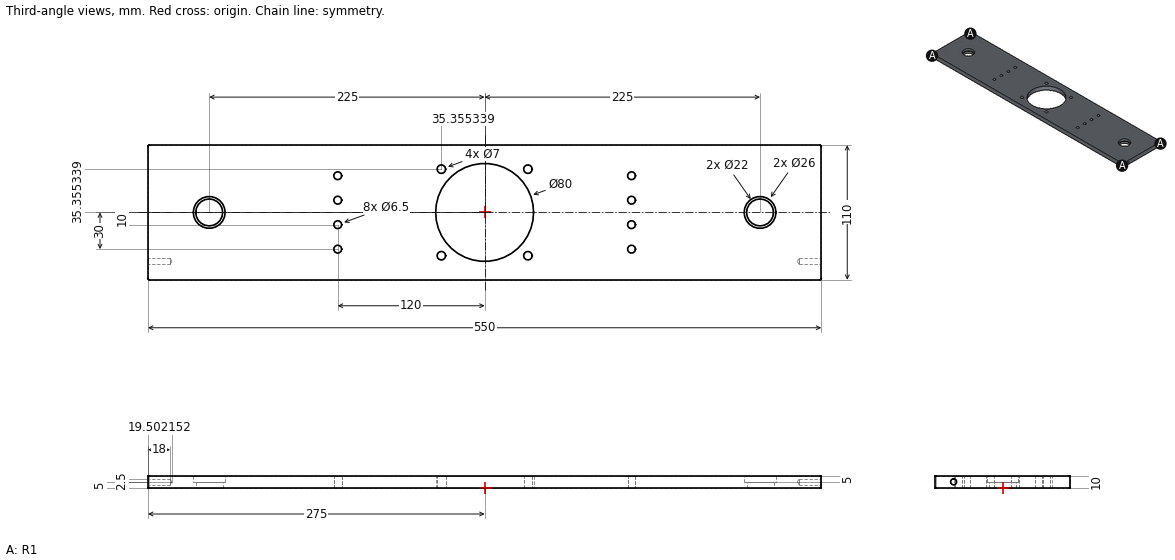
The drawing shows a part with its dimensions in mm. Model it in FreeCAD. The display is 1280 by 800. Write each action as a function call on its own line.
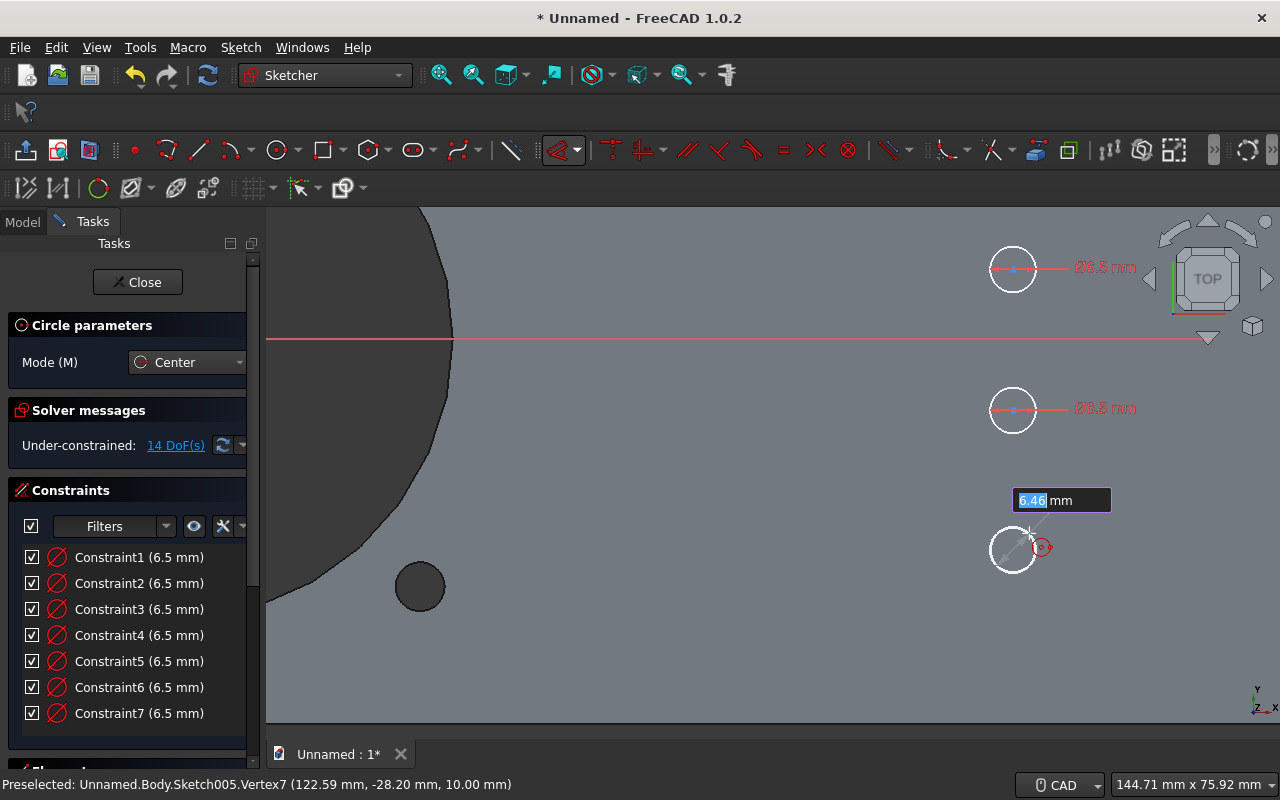
text(6.5)
key(Return)
key(Escape)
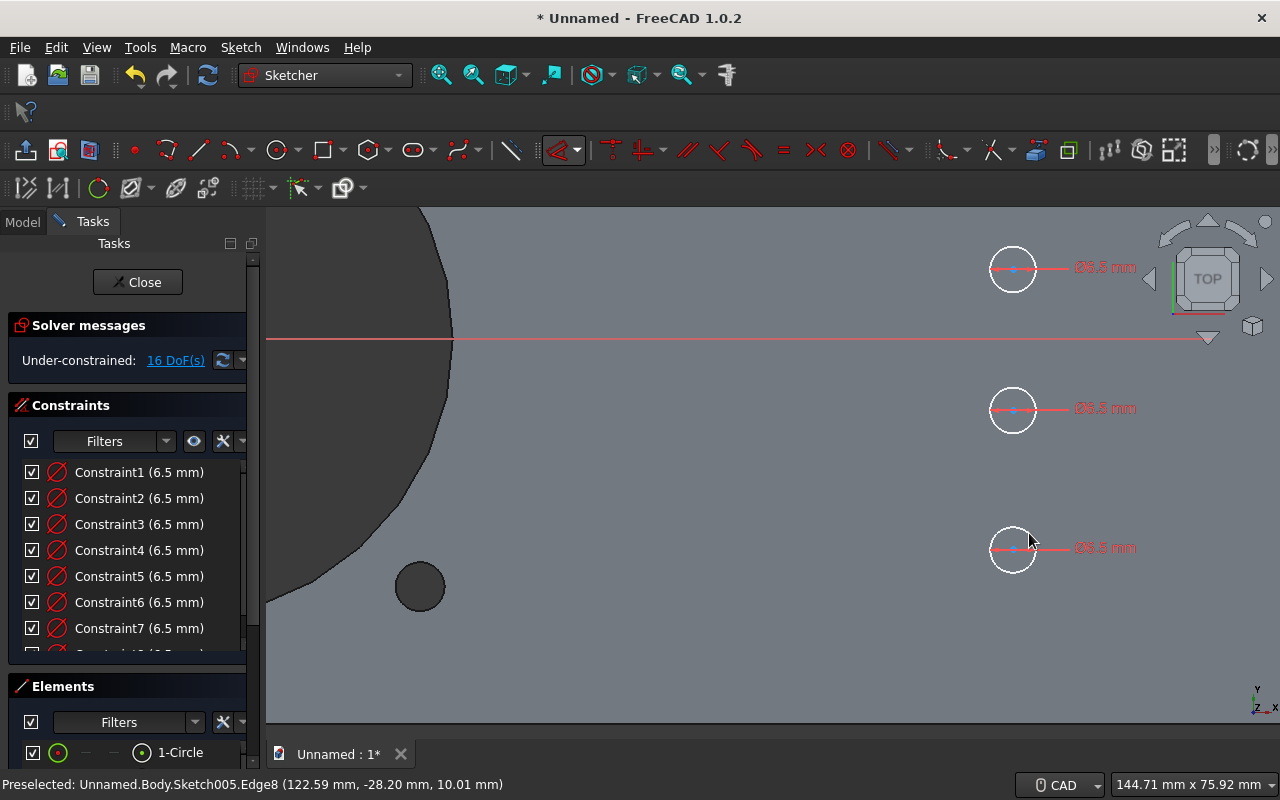
scroll(1014, 551, down, 5)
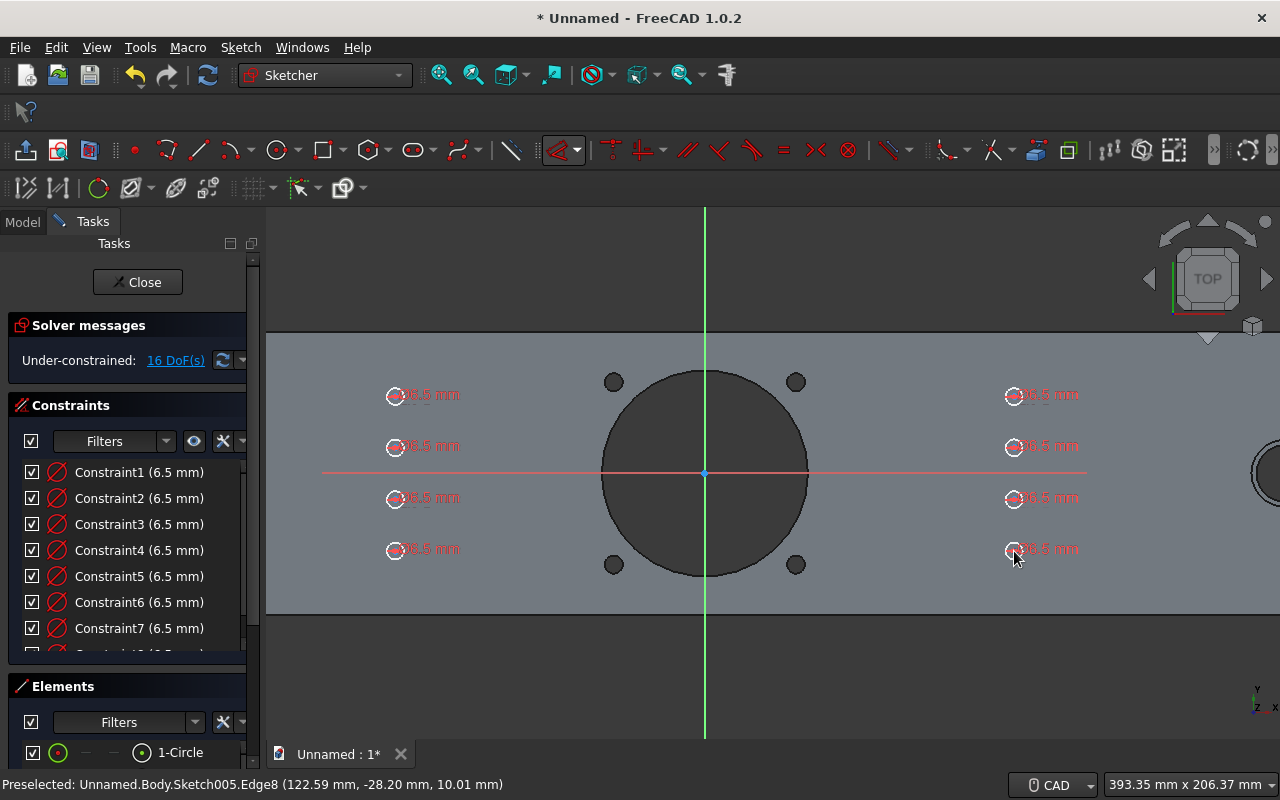
click(395, 500)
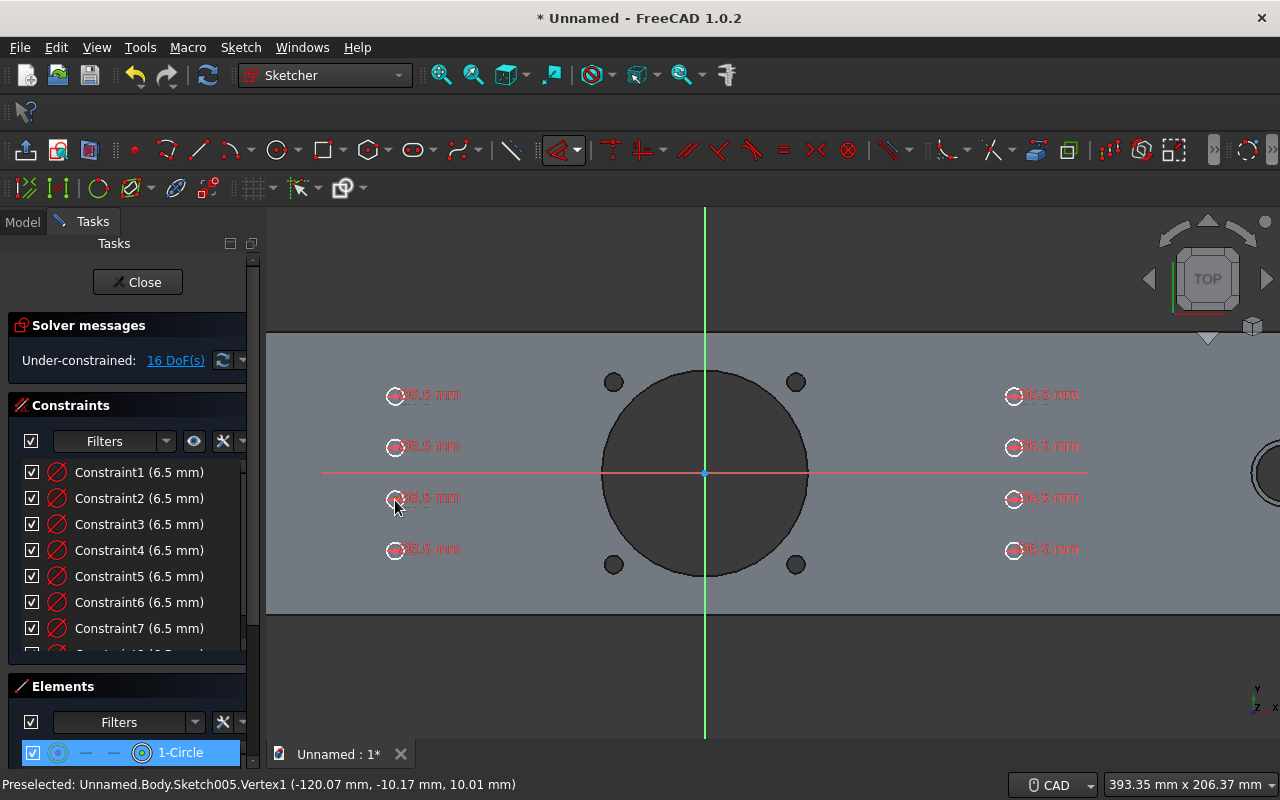
click(1014, 500)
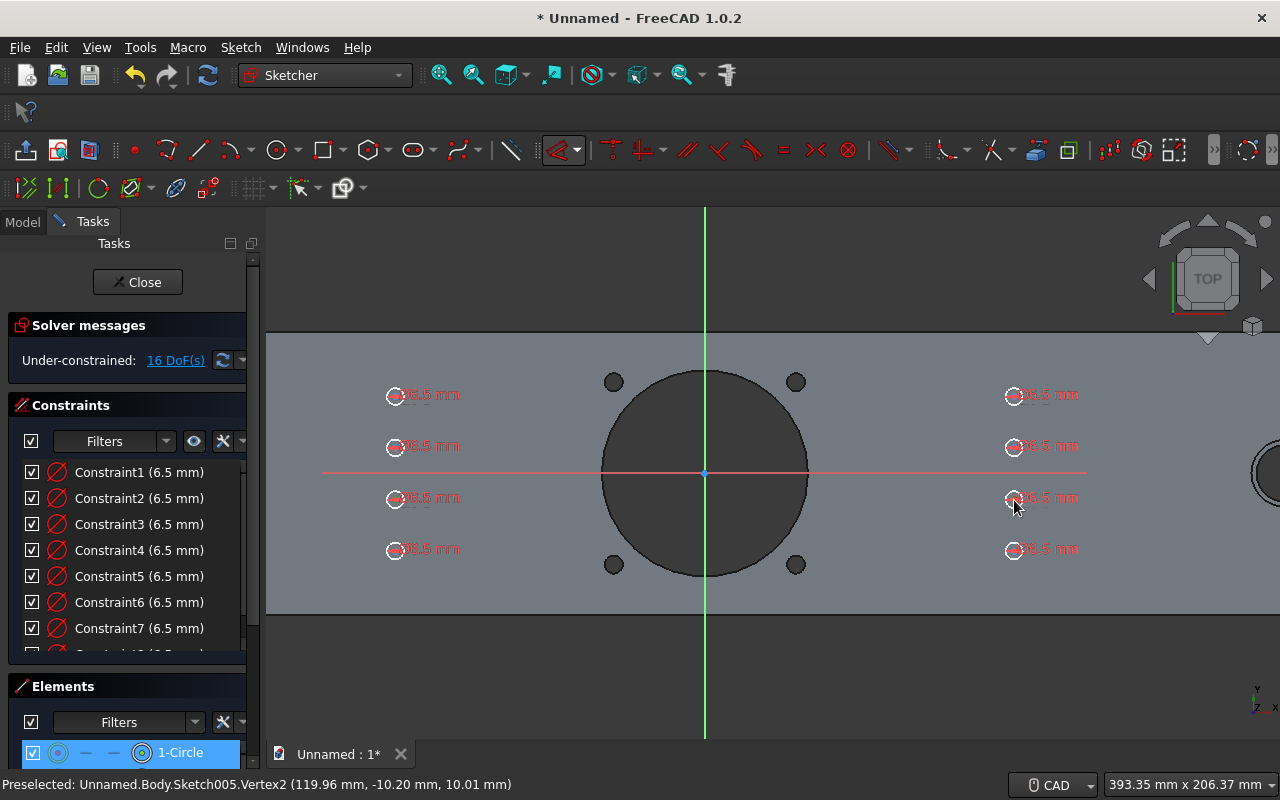
click(705, 677)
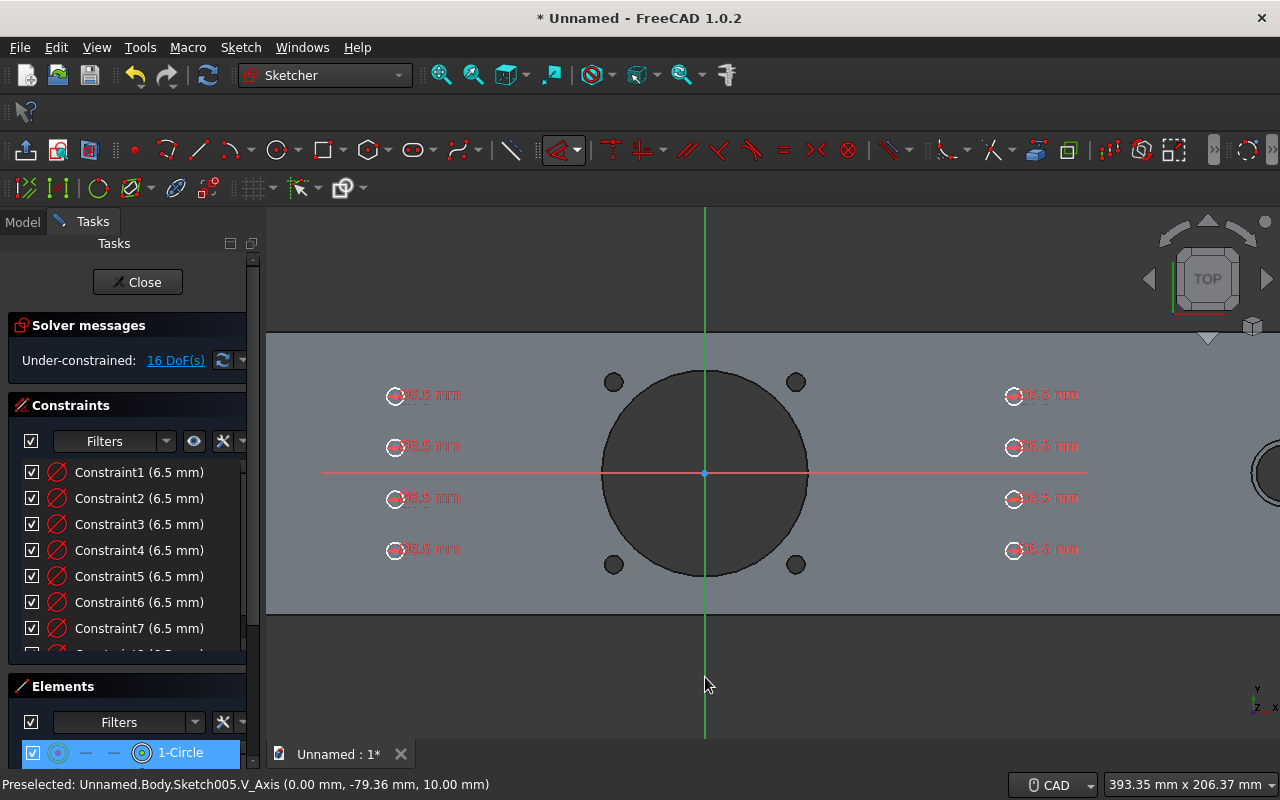
key(s)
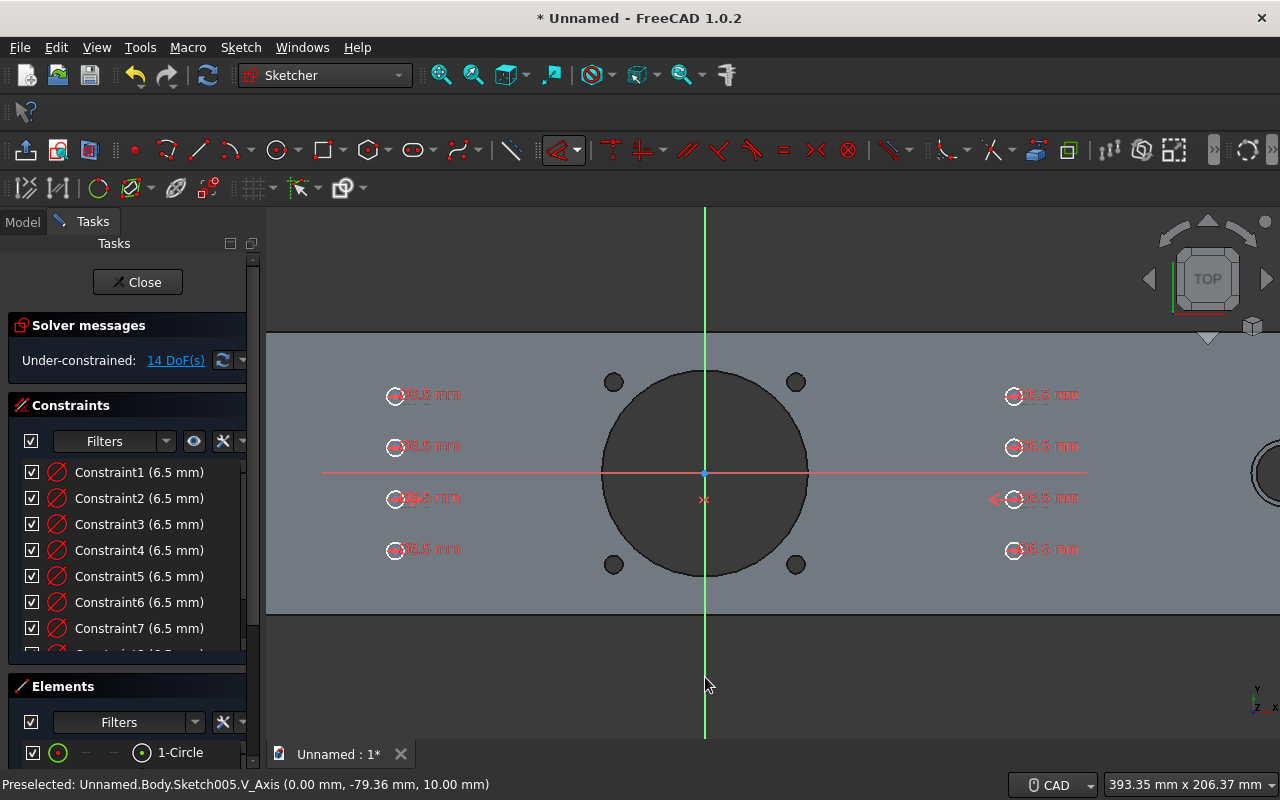
click(1014, 500)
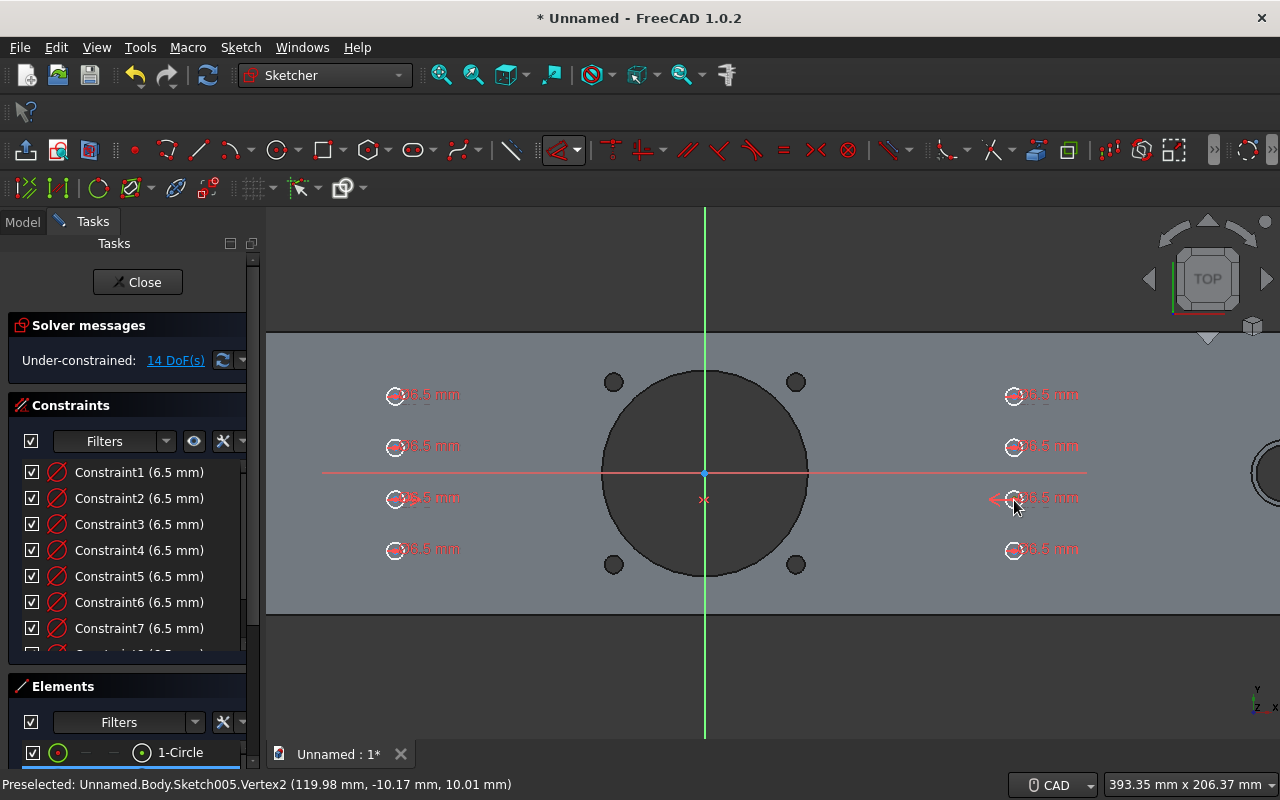
click(1014, 448)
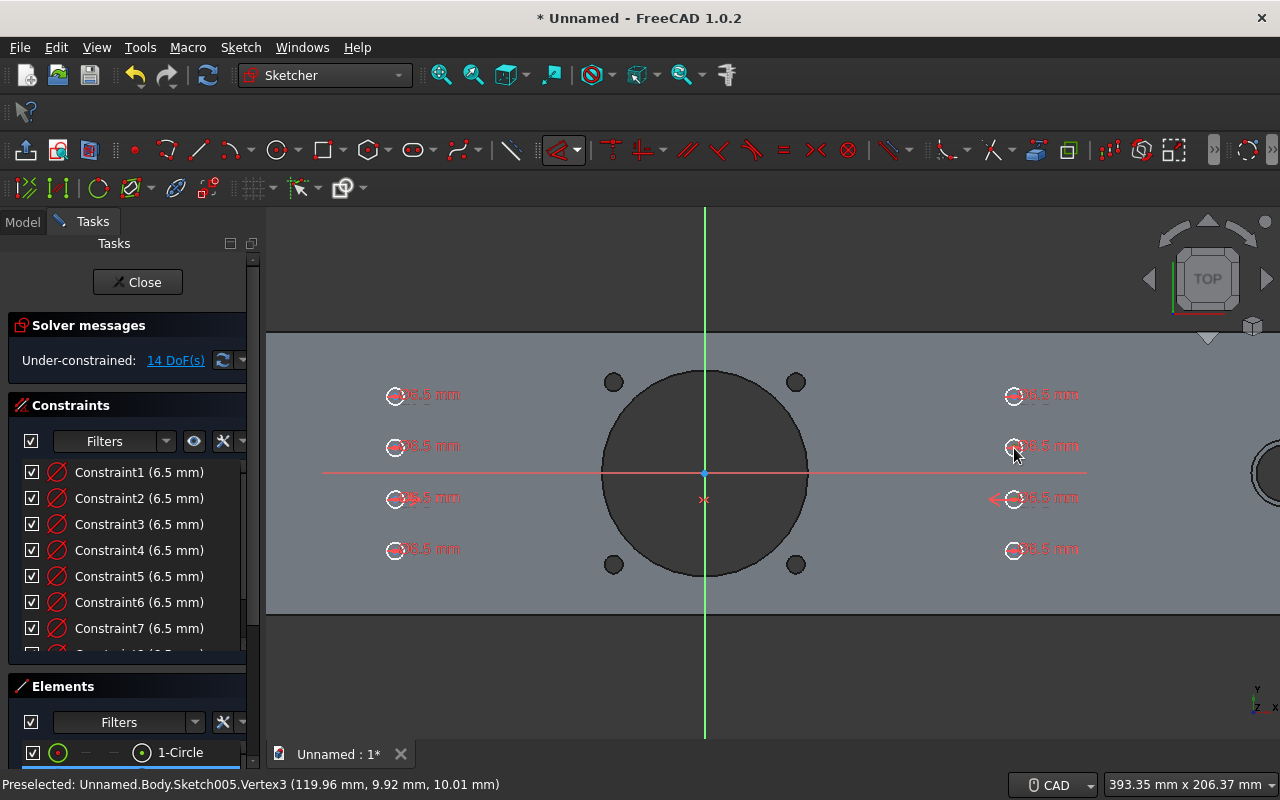
click(353, 473)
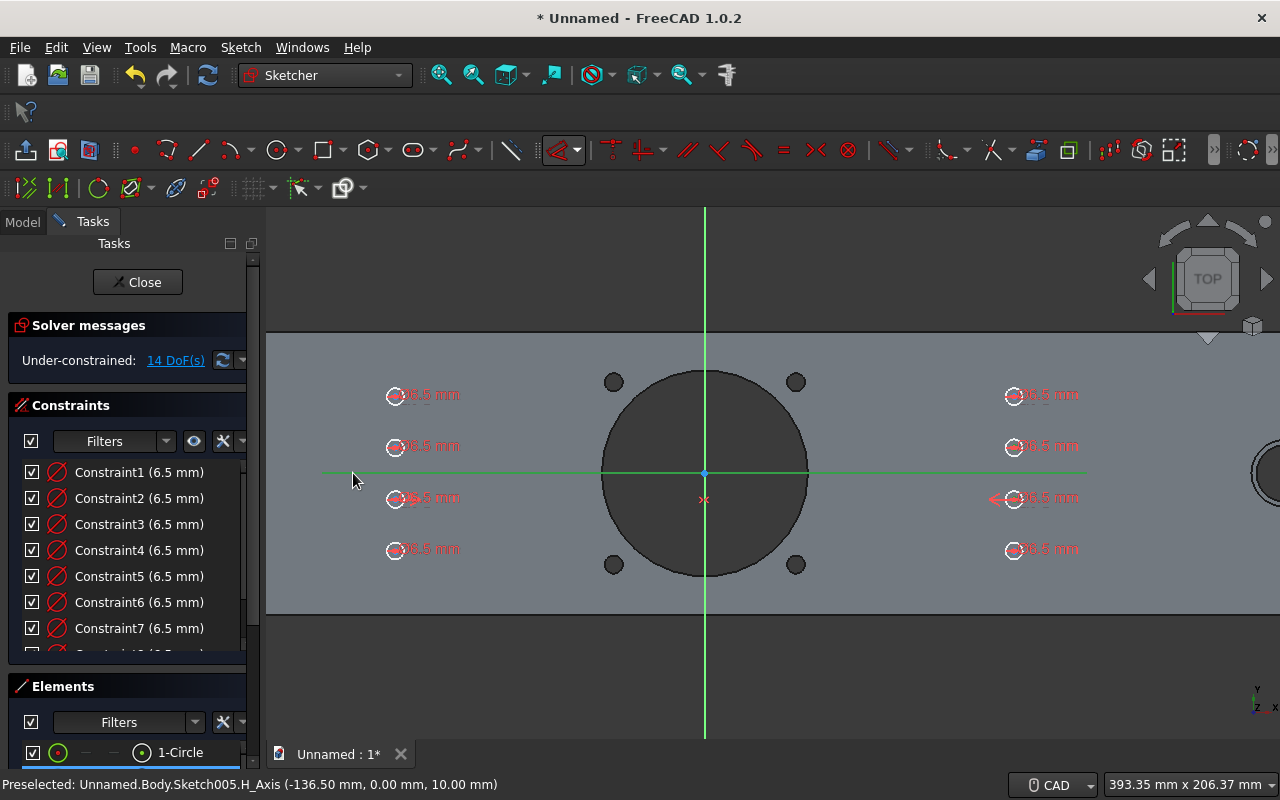
click(816, 150)